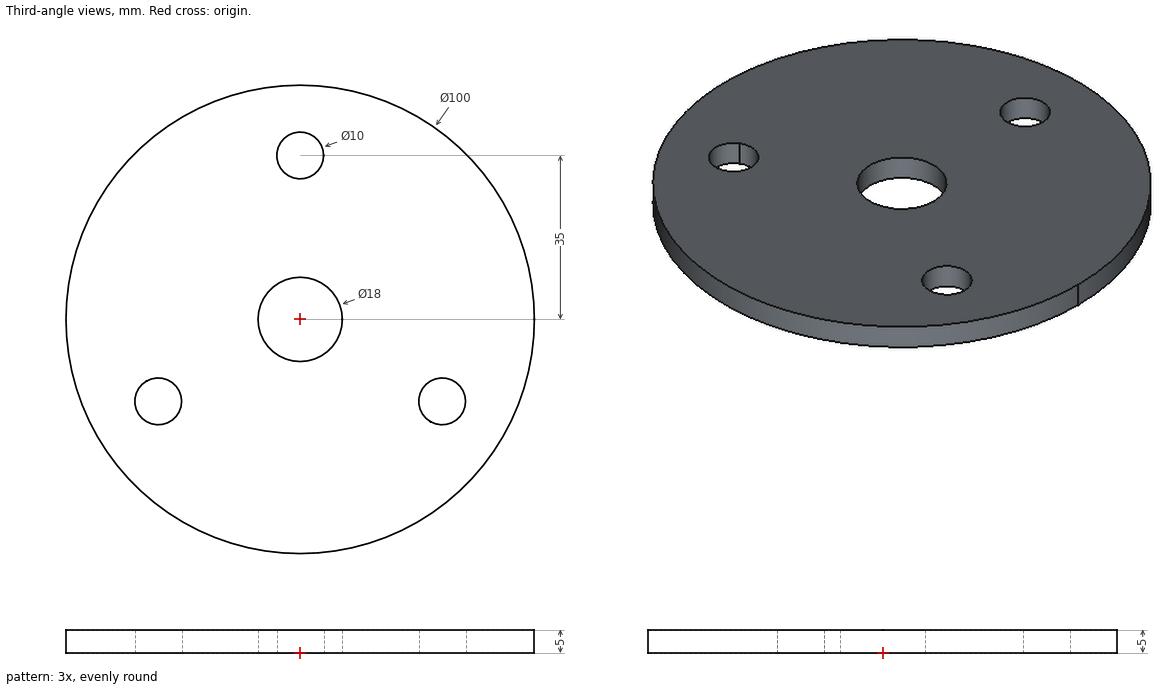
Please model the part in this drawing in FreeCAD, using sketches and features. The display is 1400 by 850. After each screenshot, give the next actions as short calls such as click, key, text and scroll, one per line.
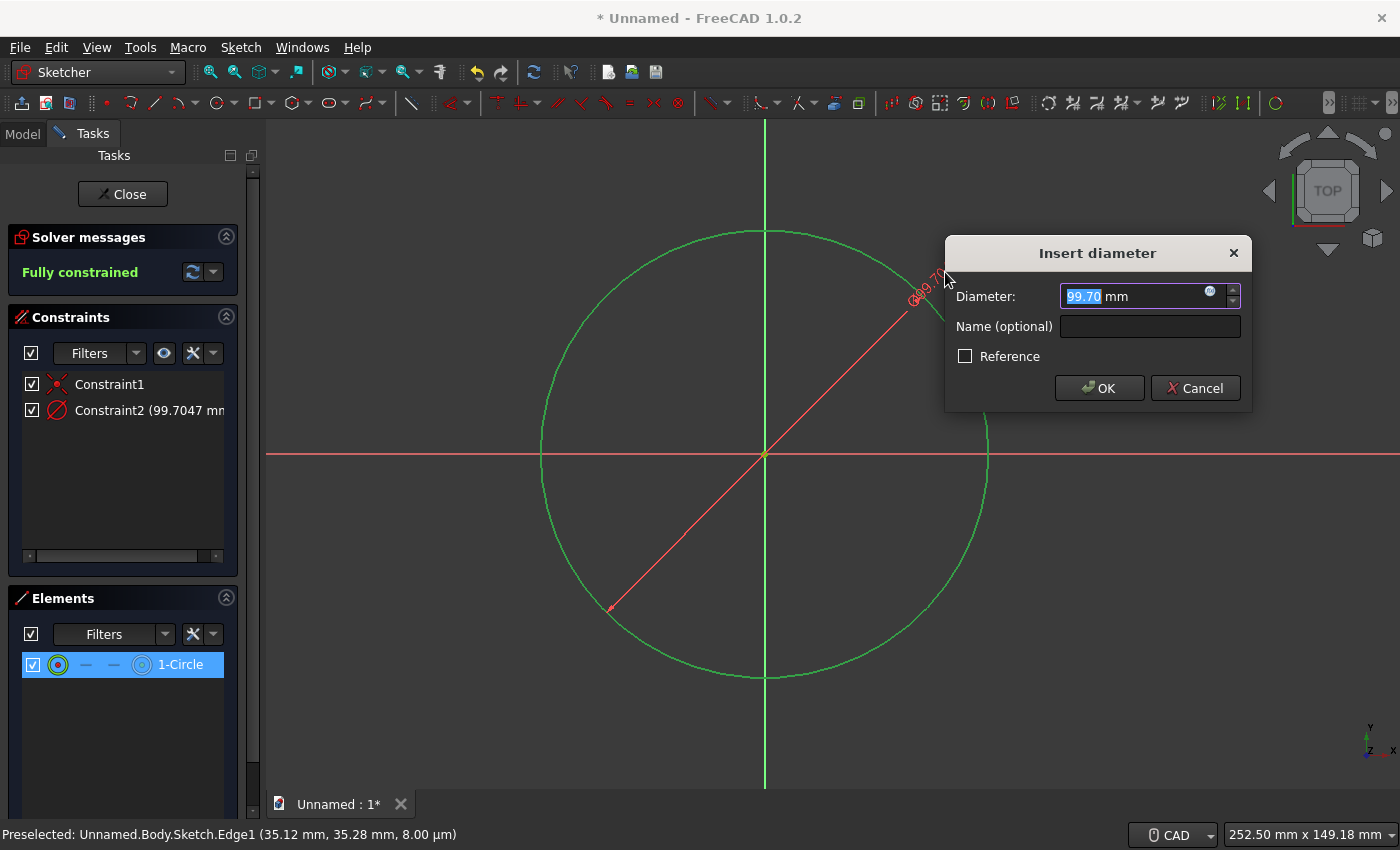
text(100)
key(Return)
key(Escape)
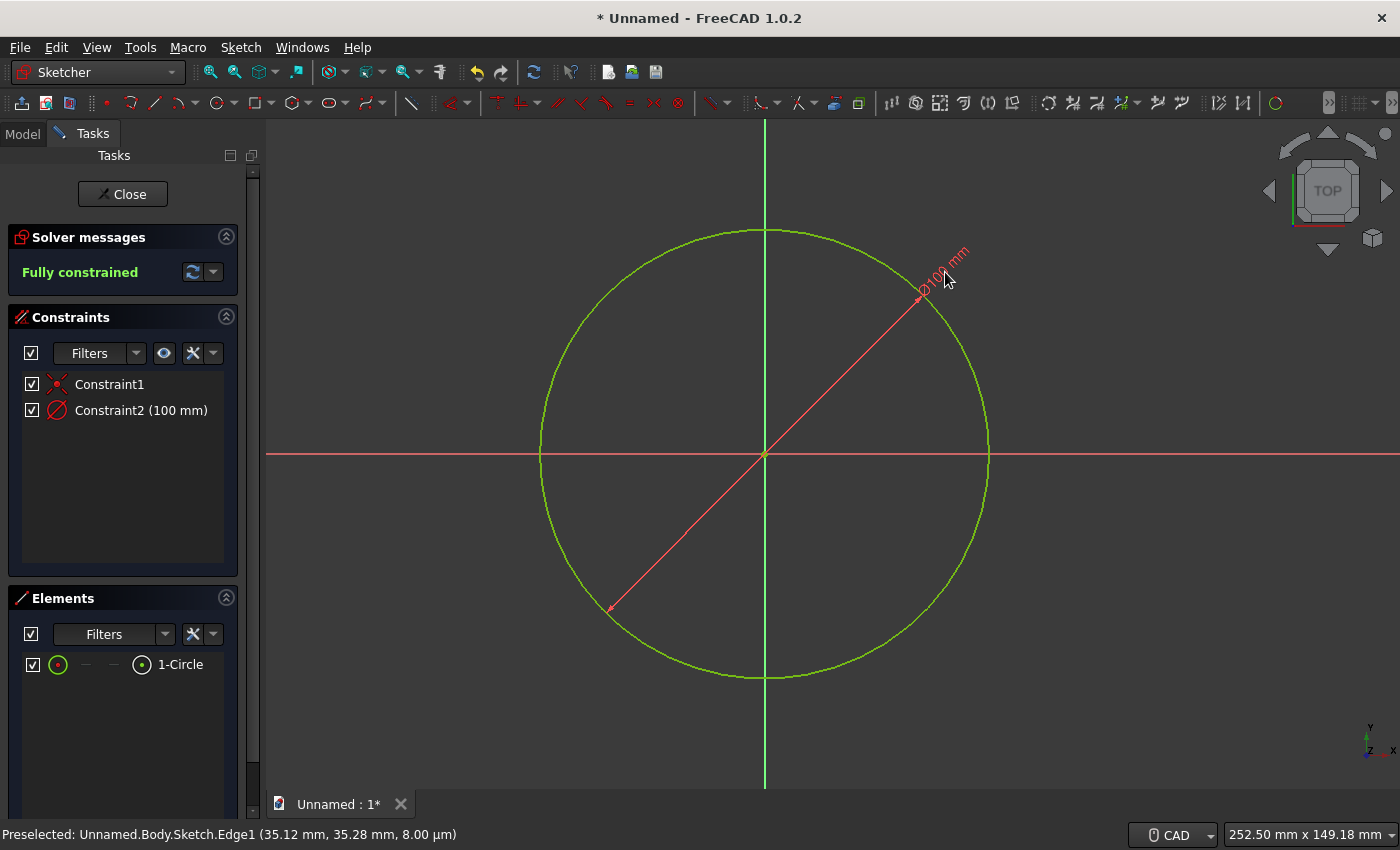
click(123, 194)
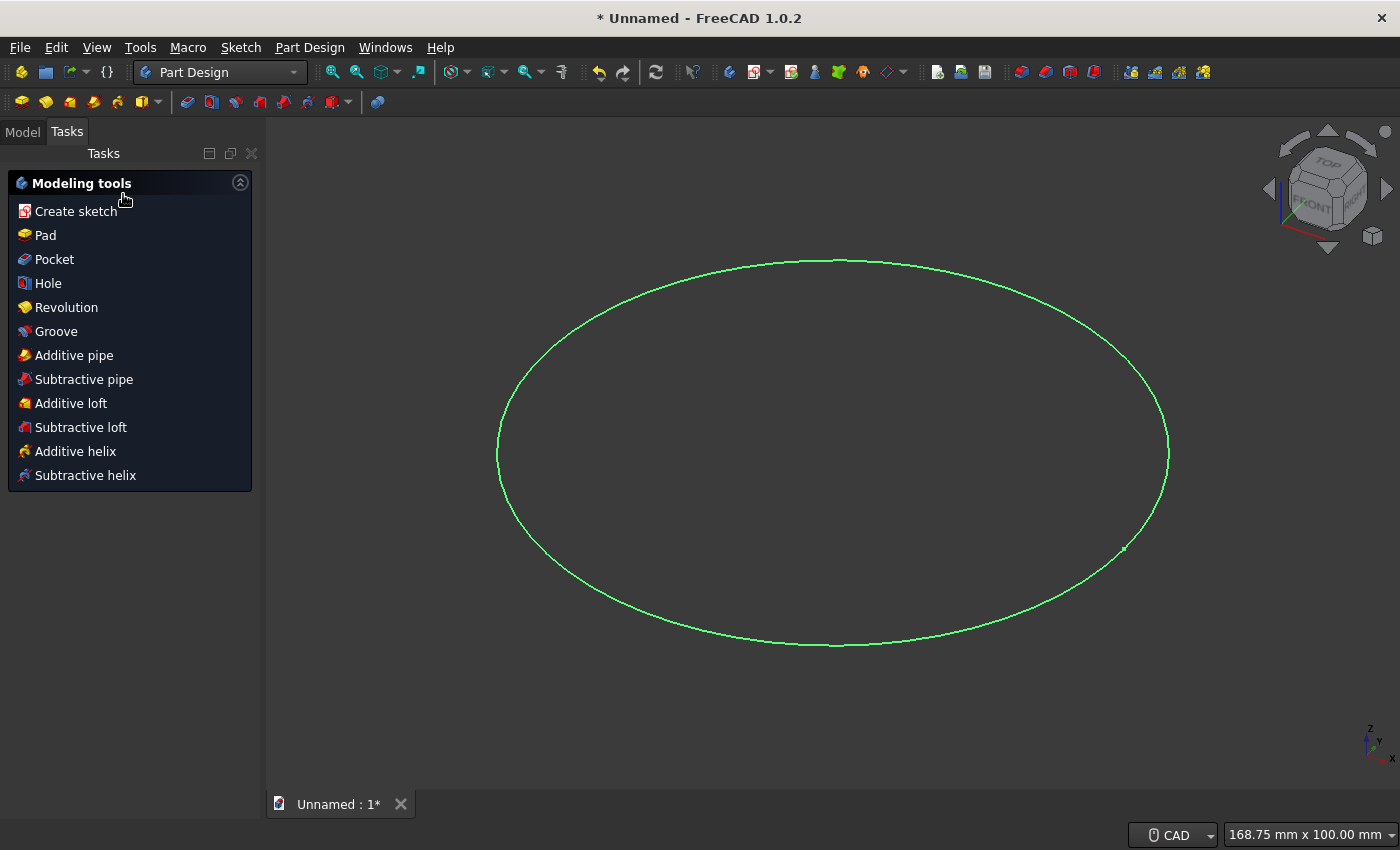
click(22, 102)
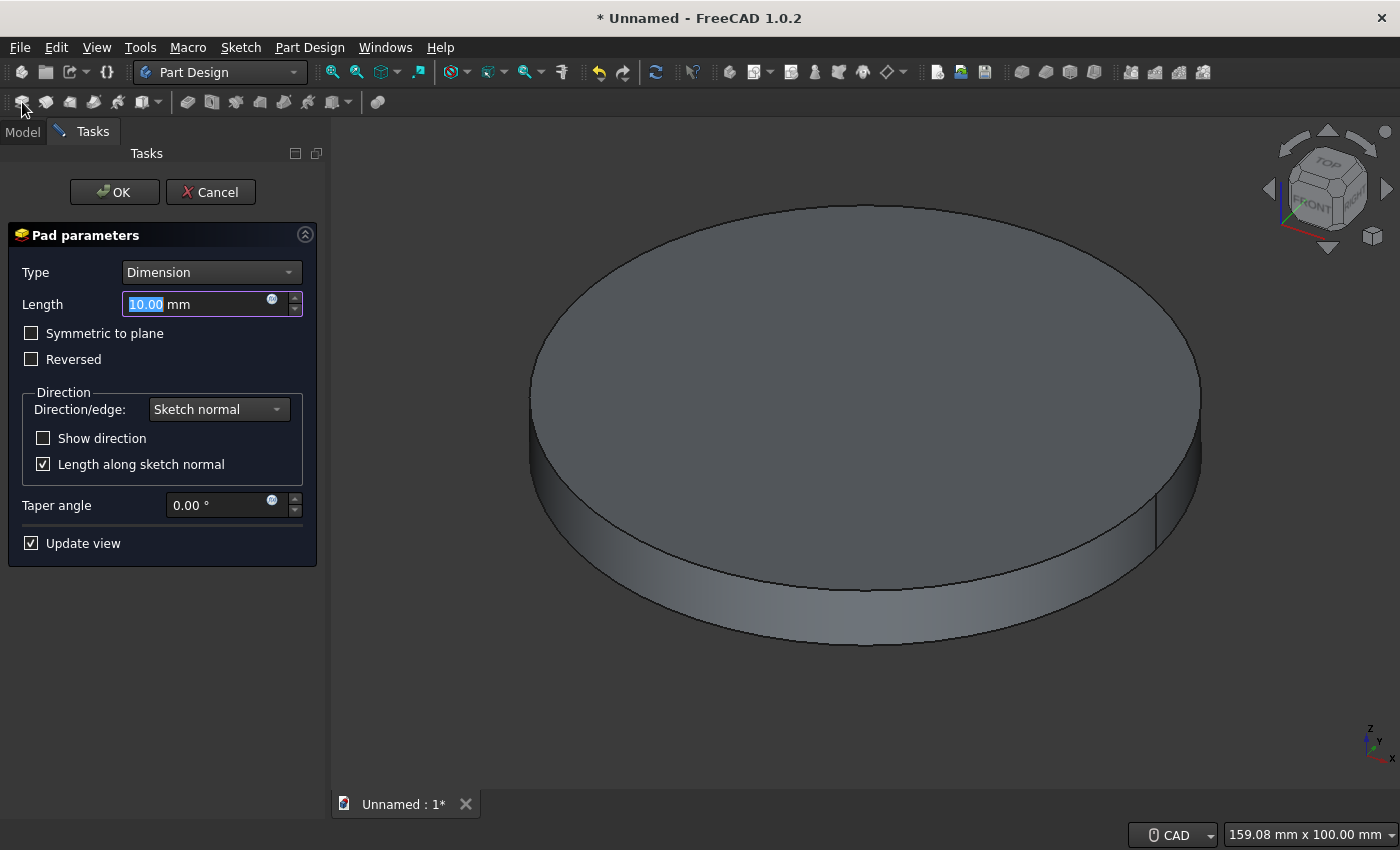
text(5)
key(Tab)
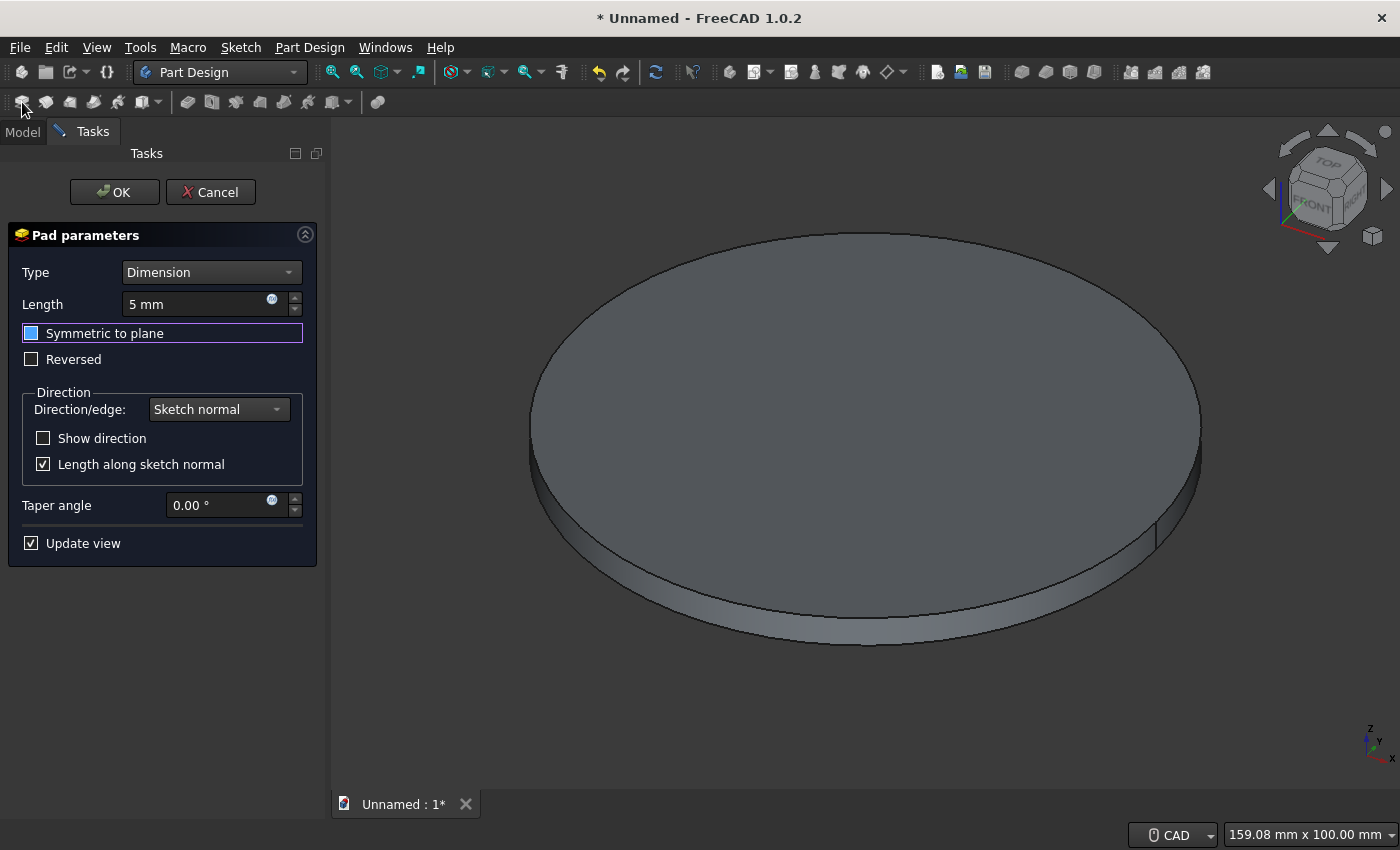
click(115, 192)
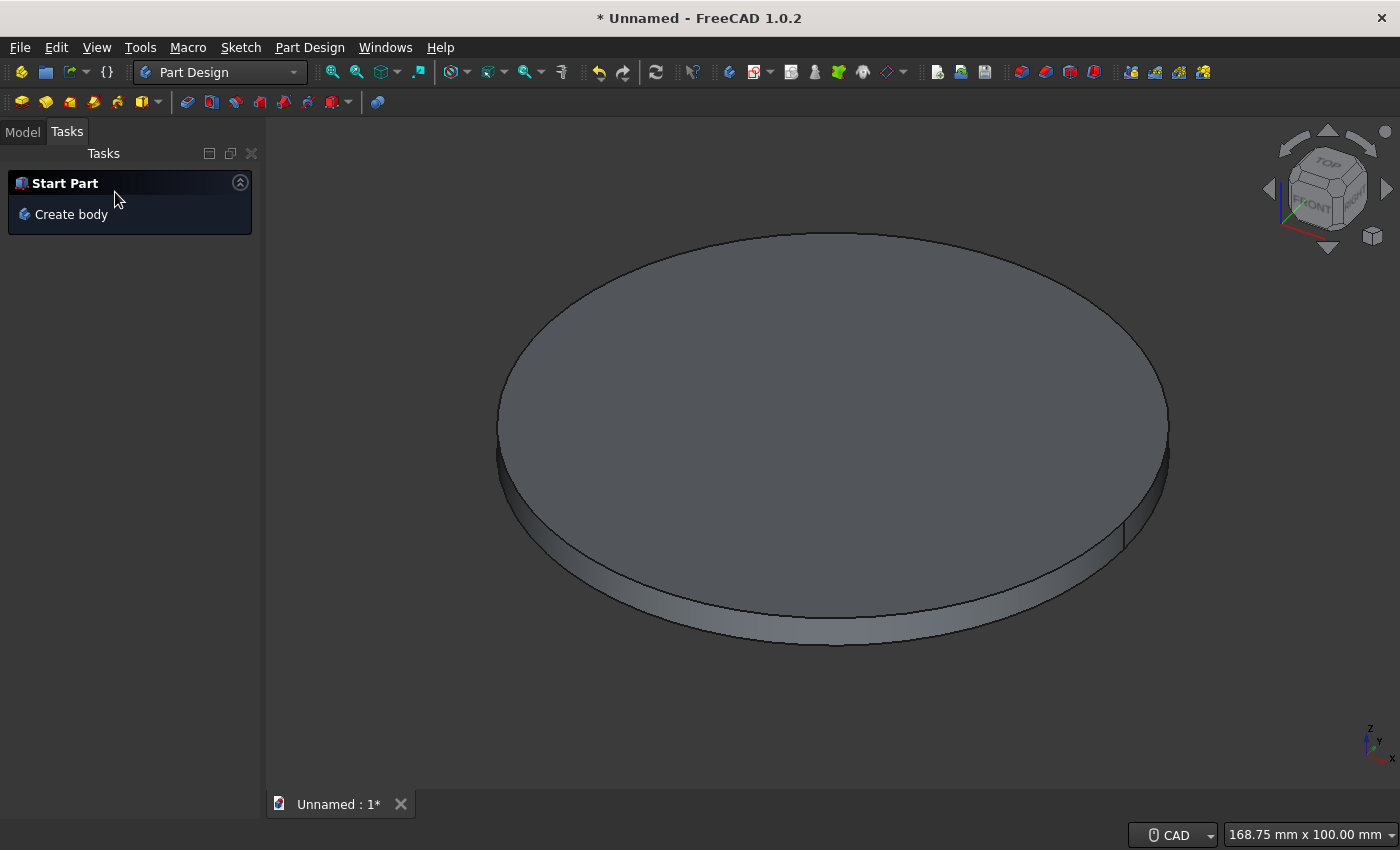
click(833, 424)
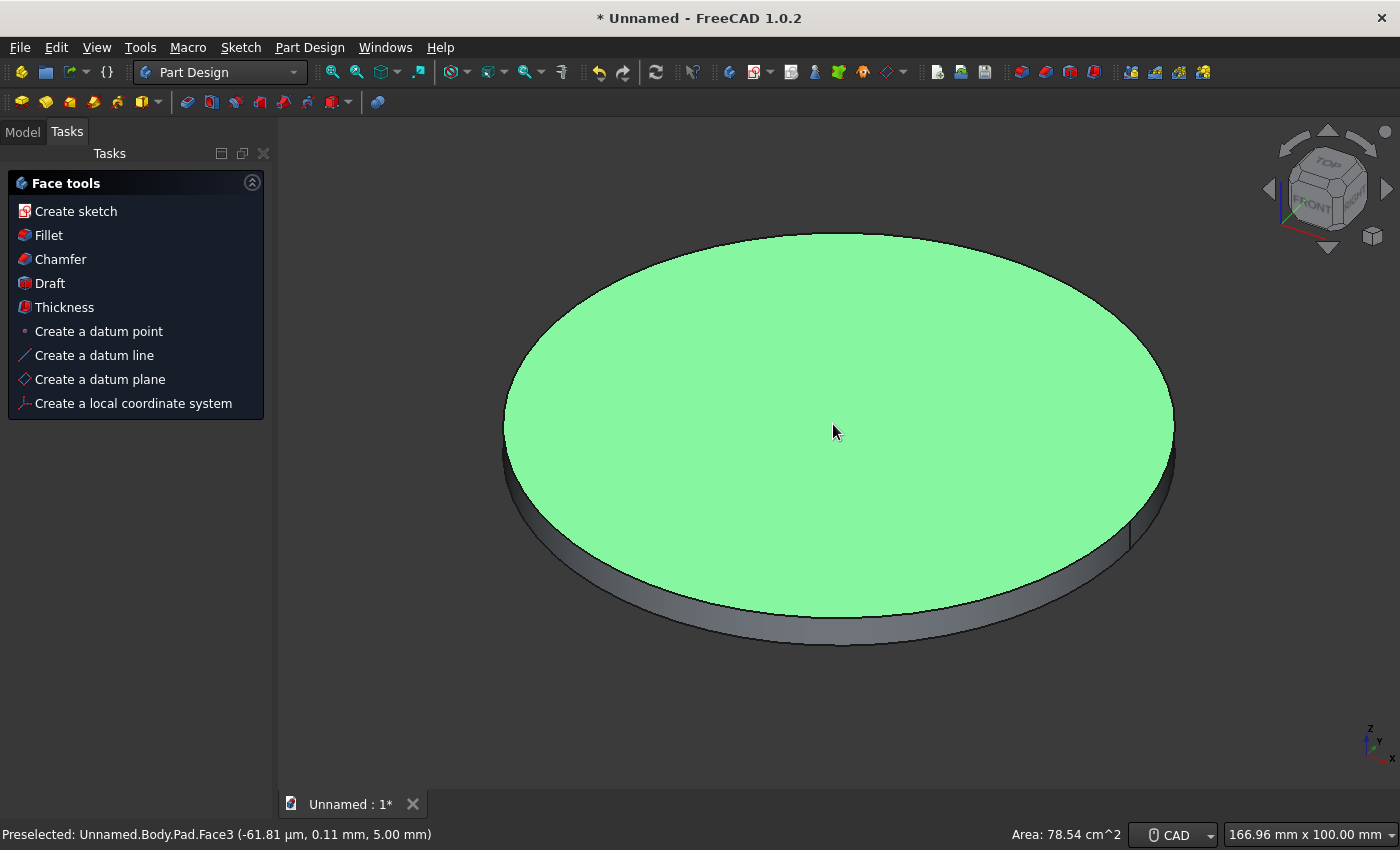
click(754, 72)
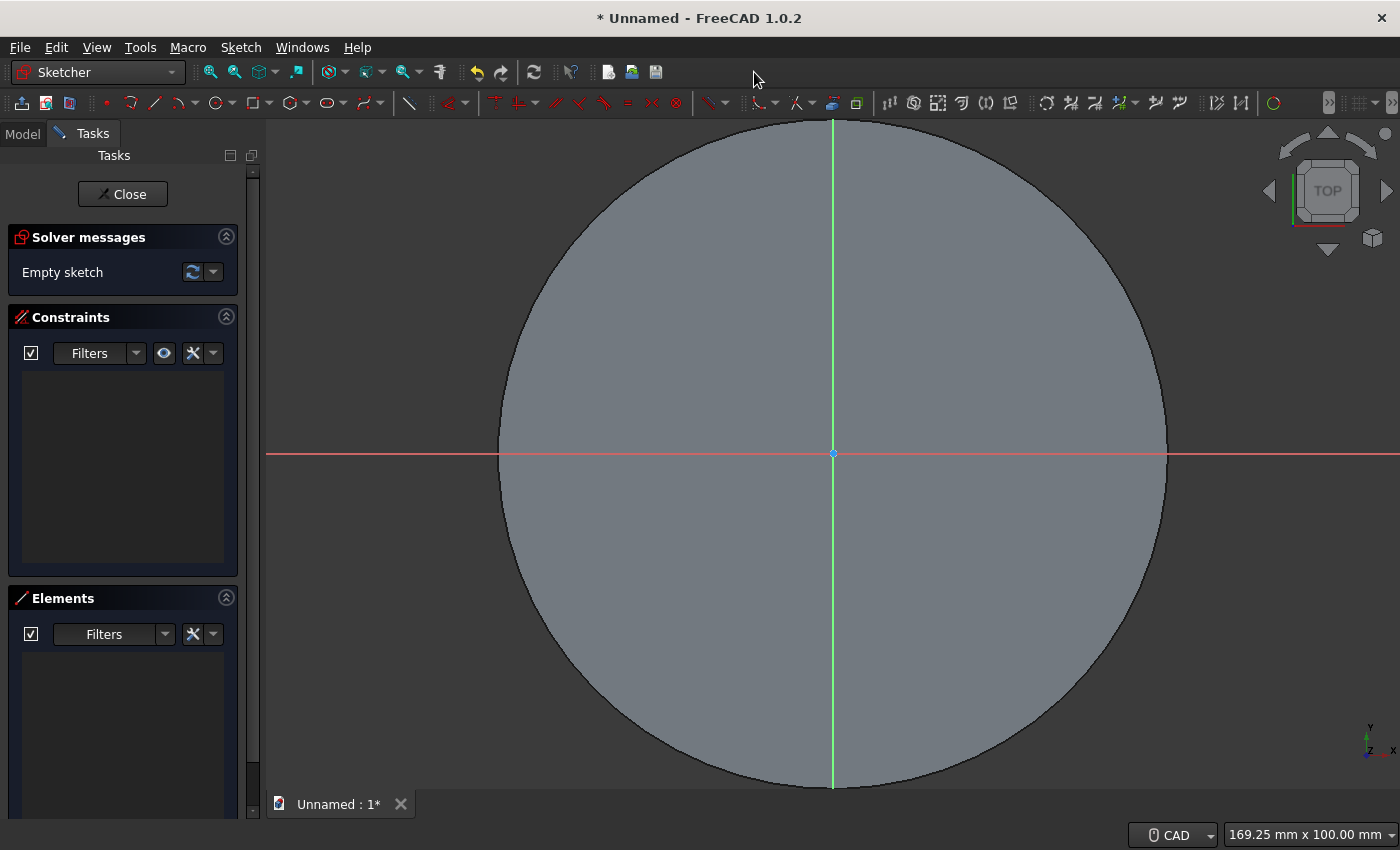
scroll(847, 173, up, 9)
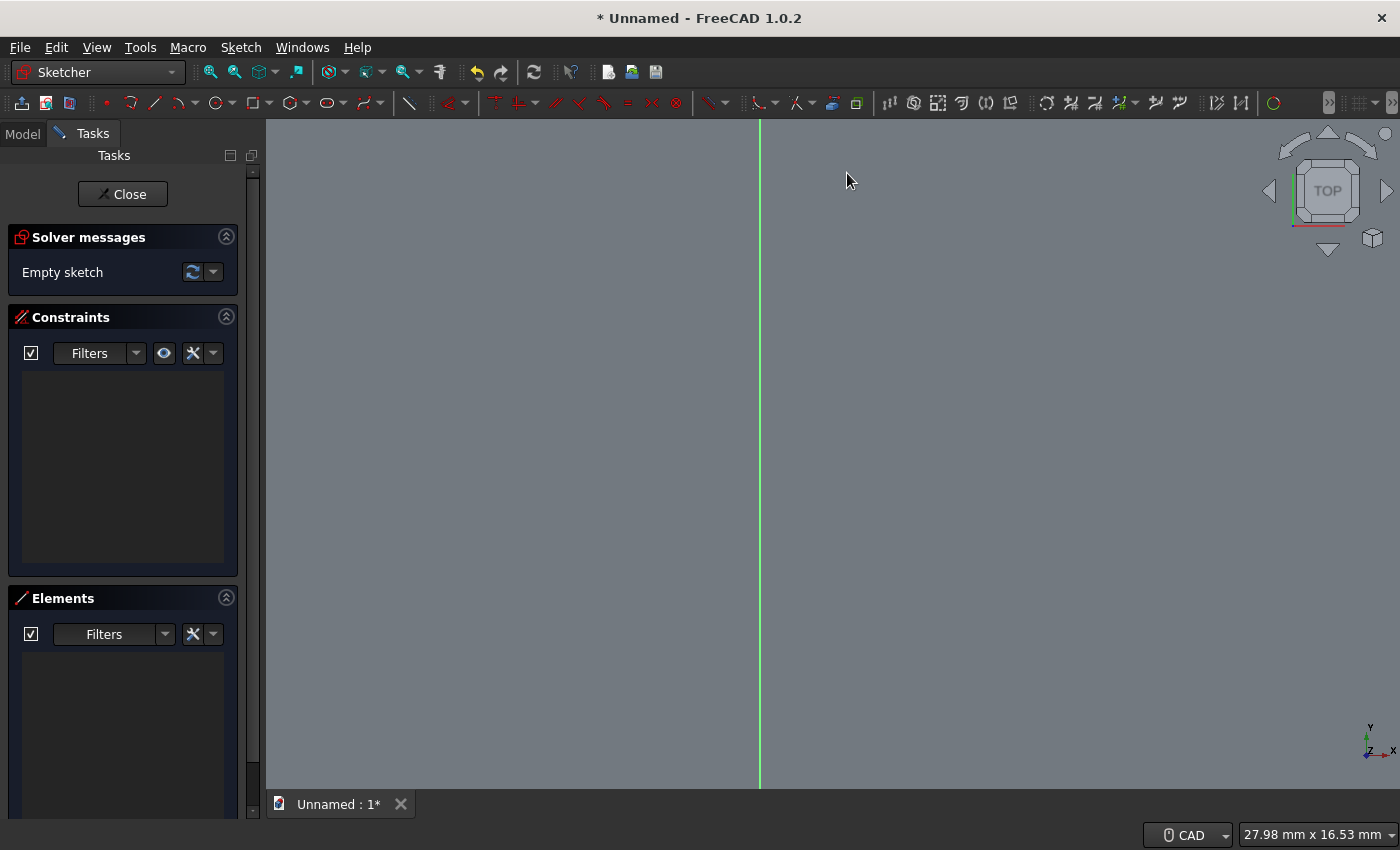
click(216, 104)